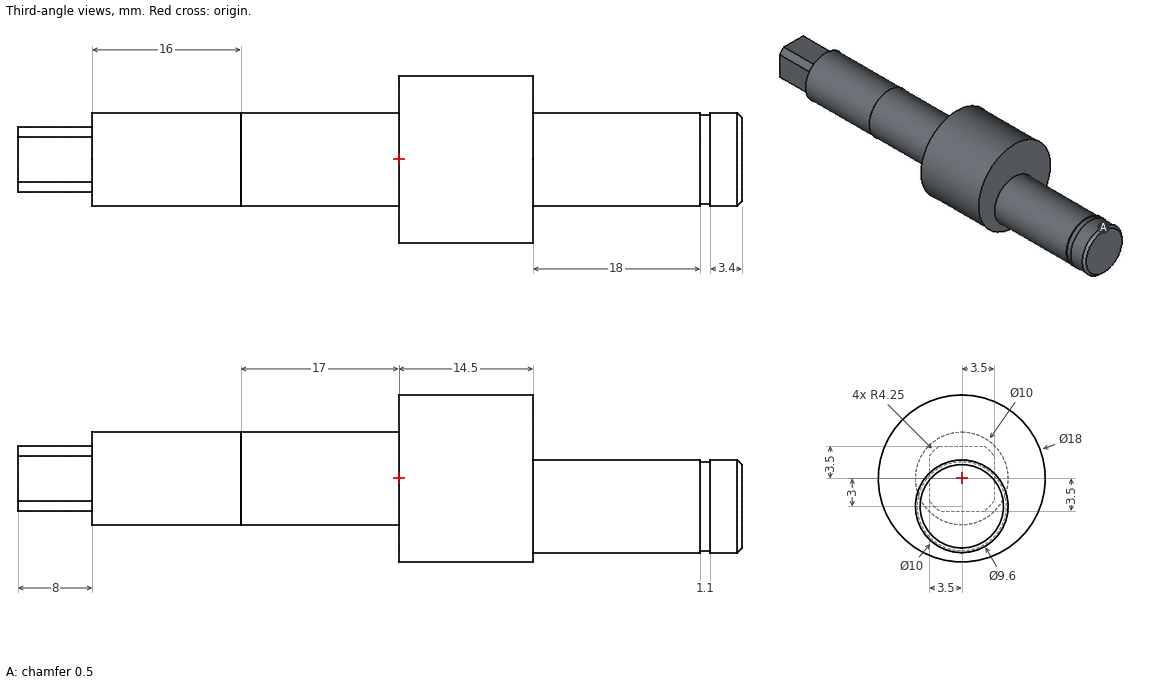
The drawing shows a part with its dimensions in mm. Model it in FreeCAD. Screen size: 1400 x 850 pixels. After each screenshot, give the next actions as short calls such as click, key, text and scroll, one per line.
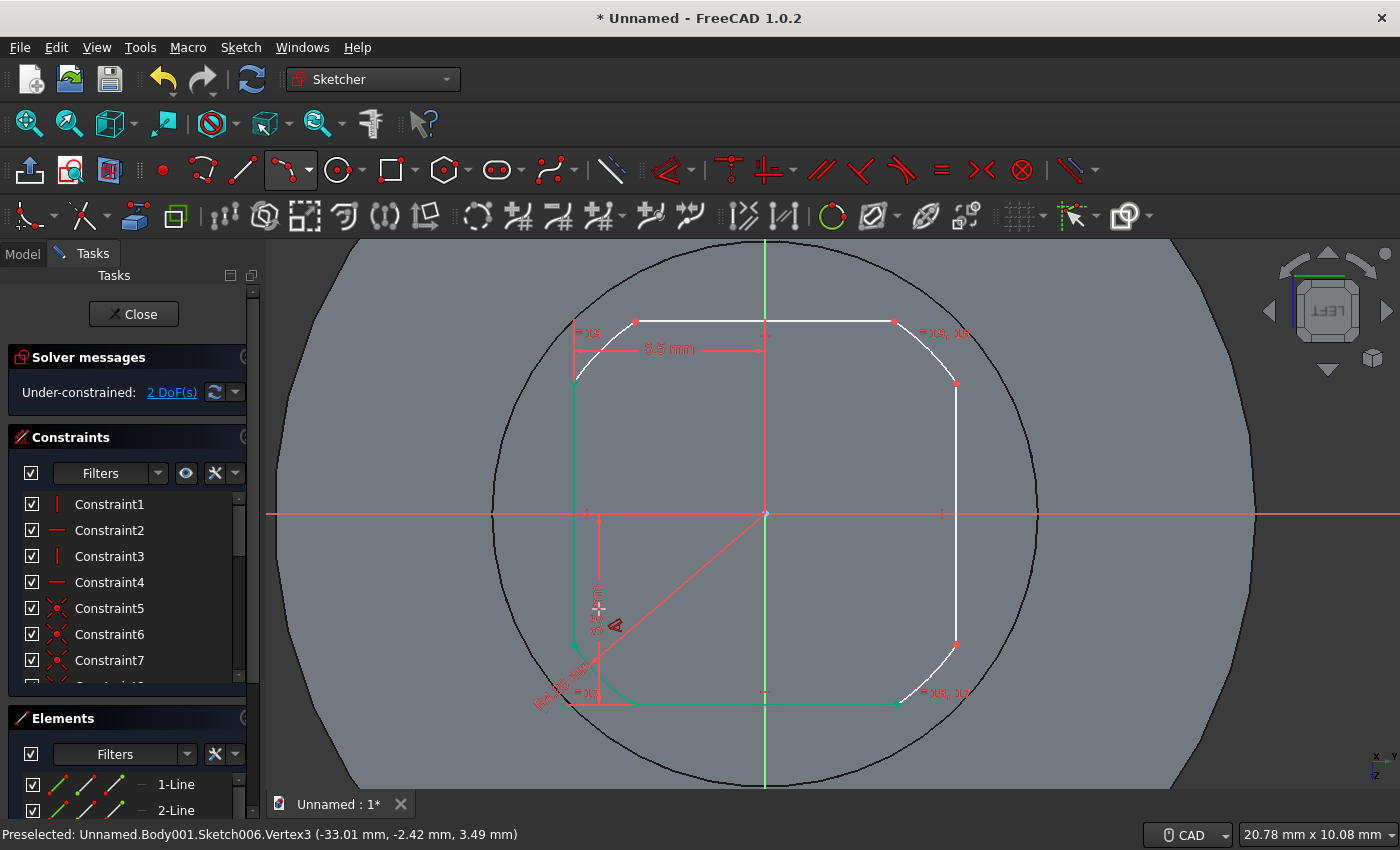
click(956, 645)
click(861, 679)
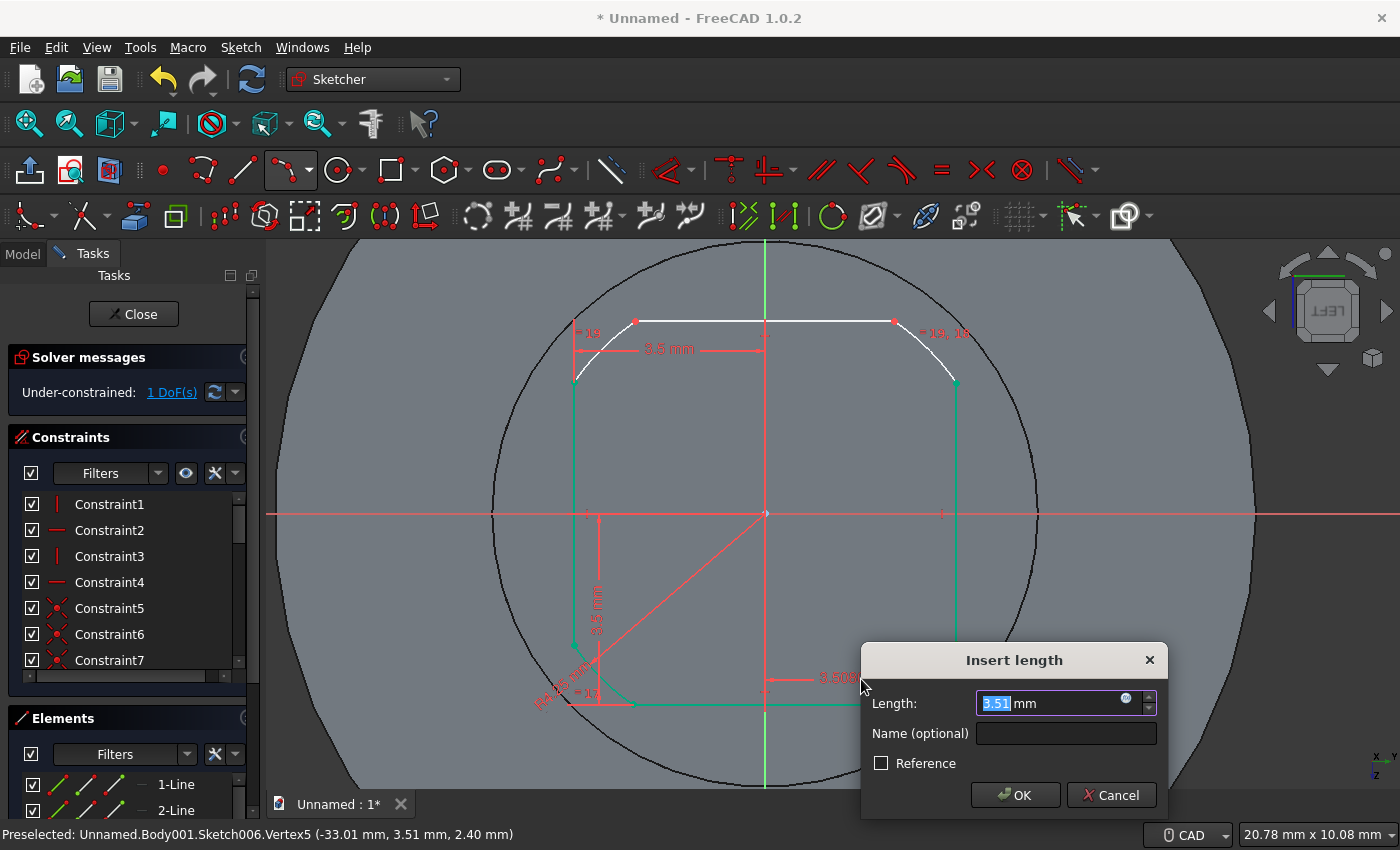
text(3.5)
key(Return)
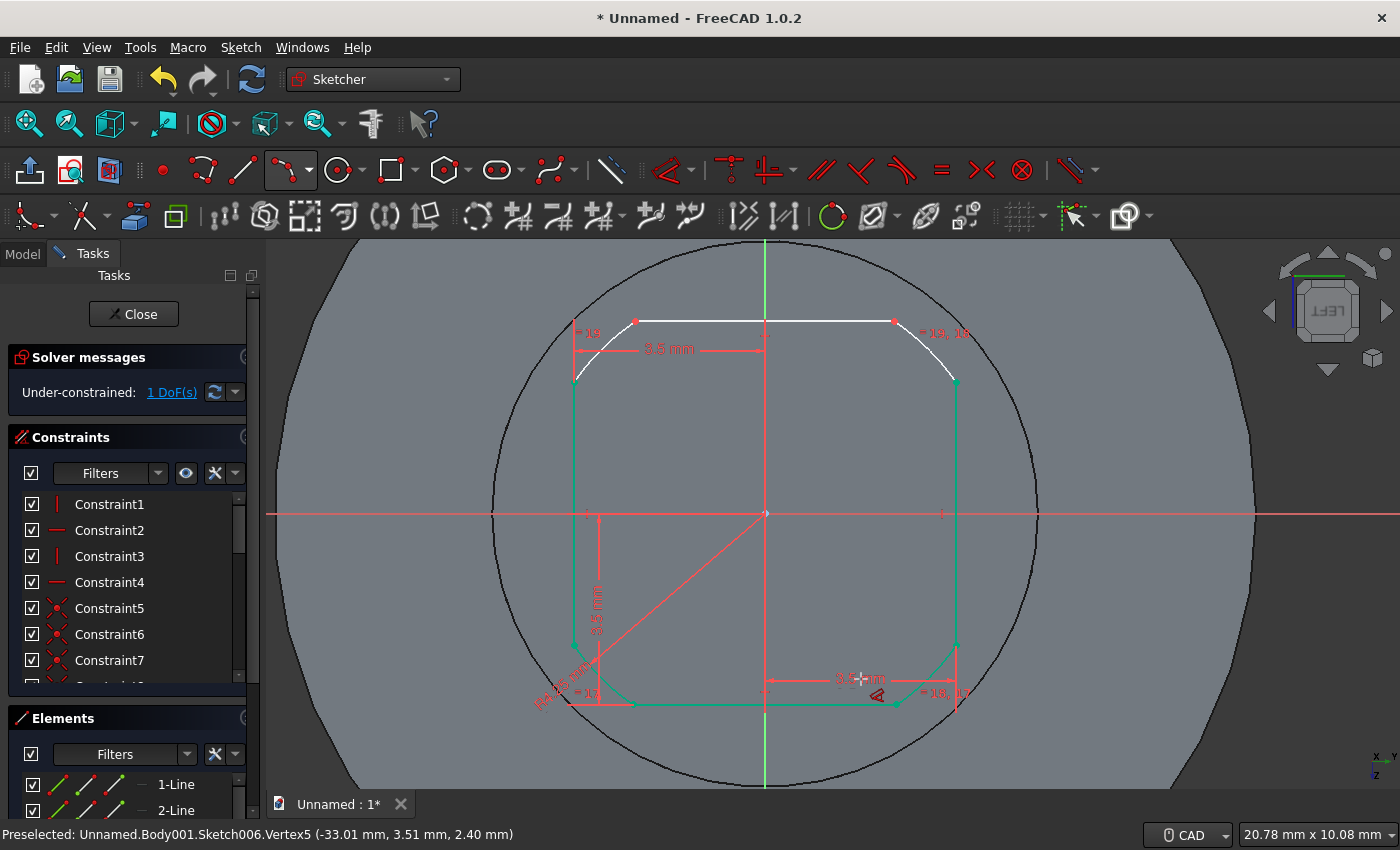
click(894, 321)
click(928, 418)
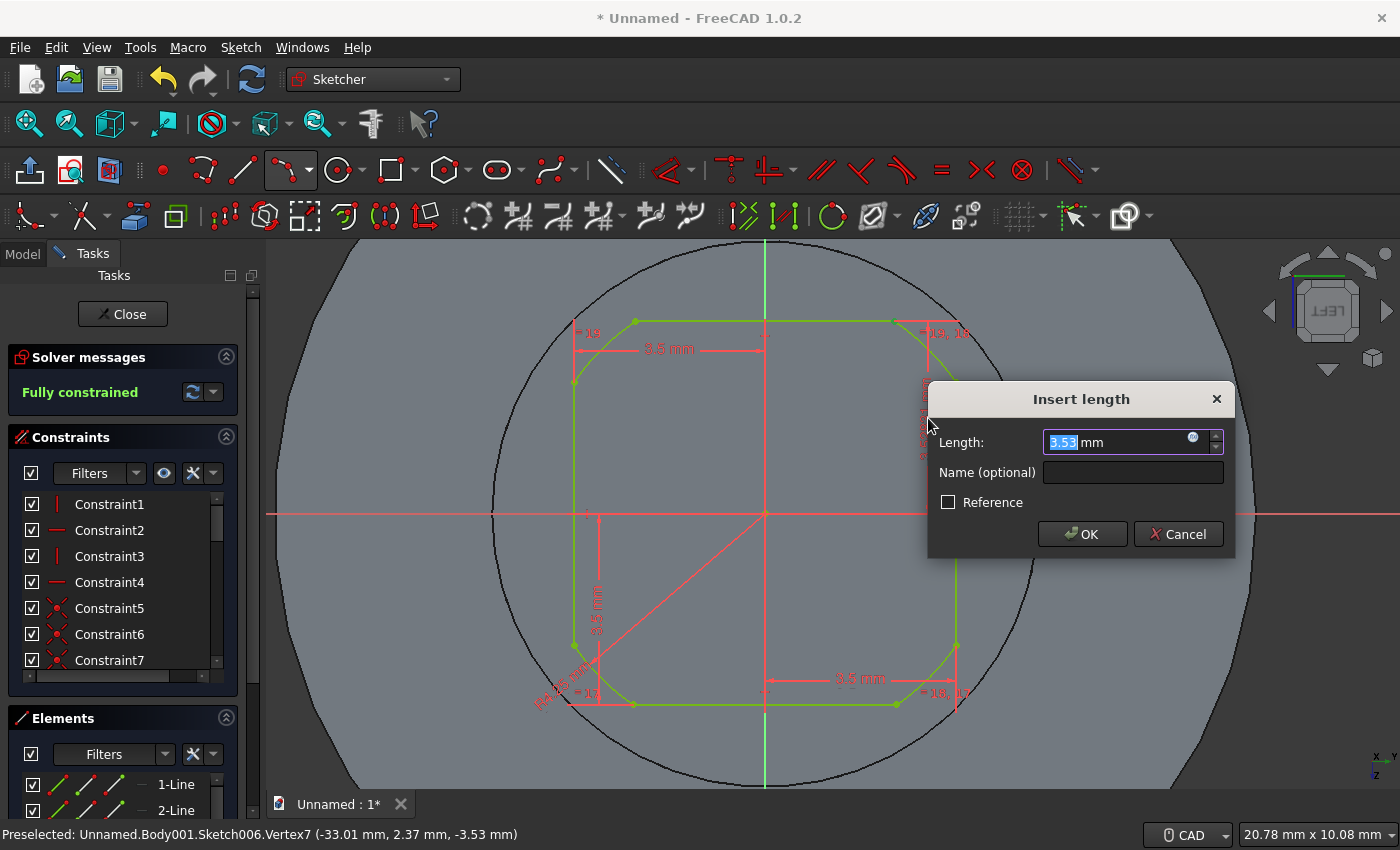
text(3.5)
key(Return)
key(Escape)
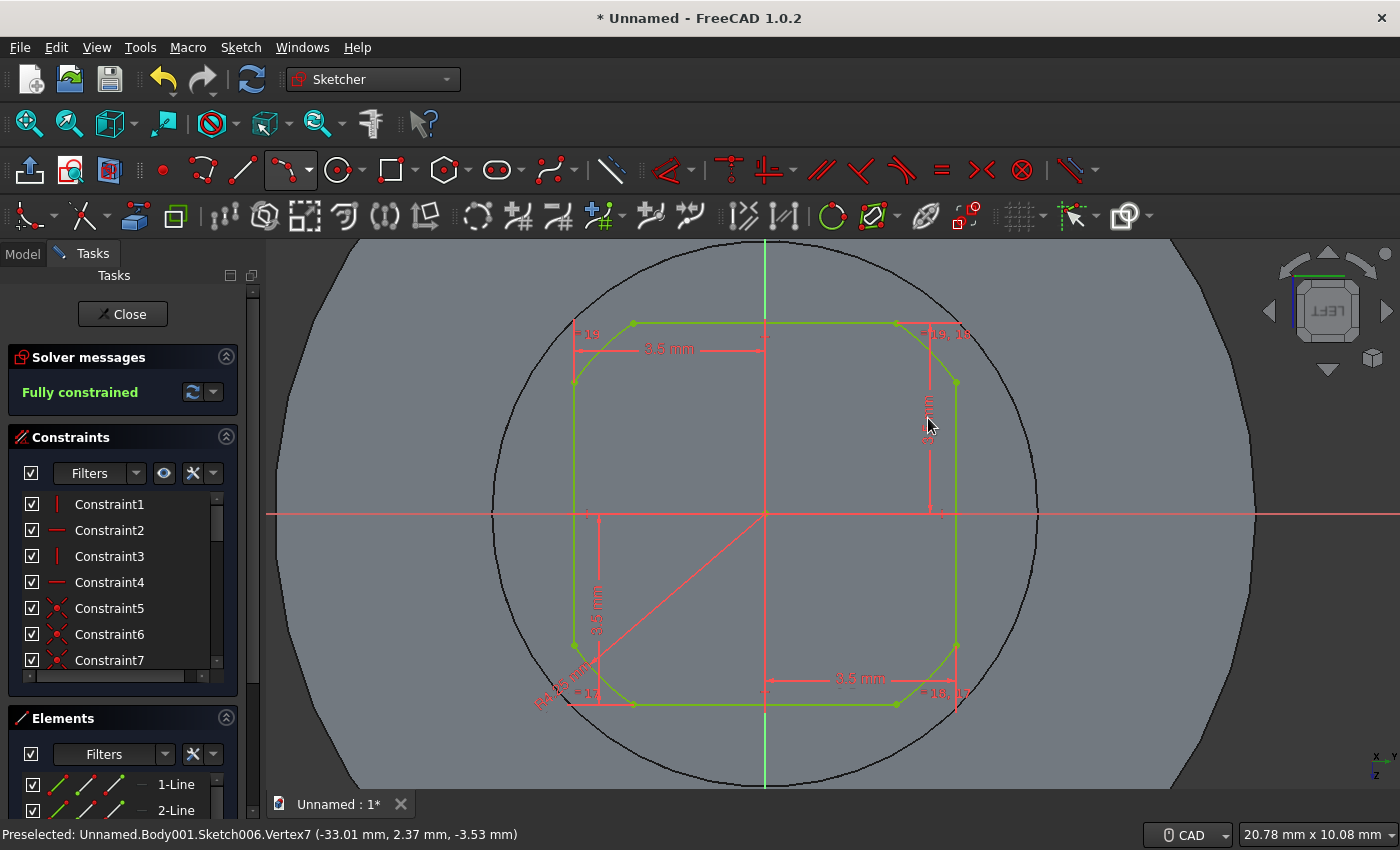
click(123, 314)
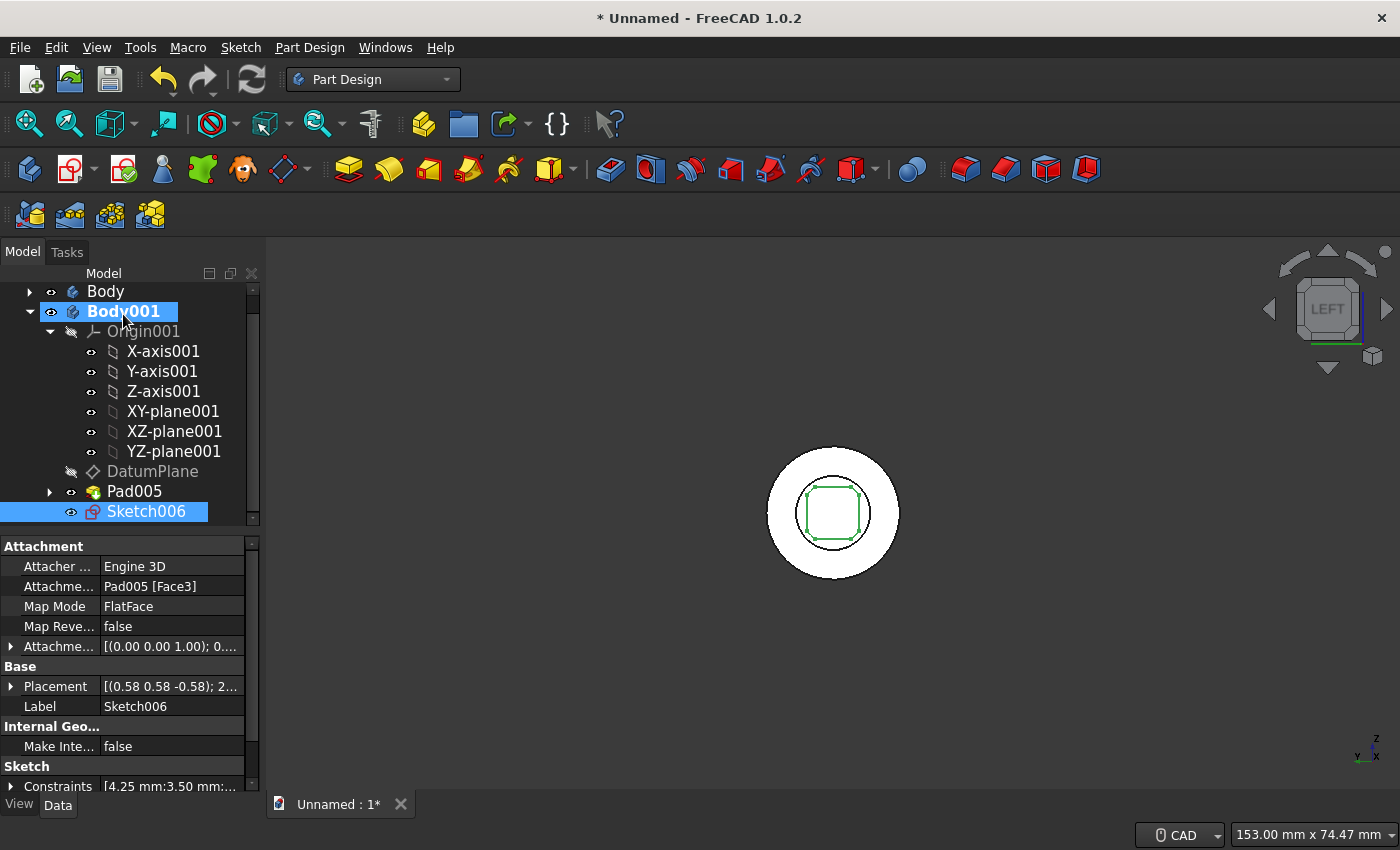
click(350, 170)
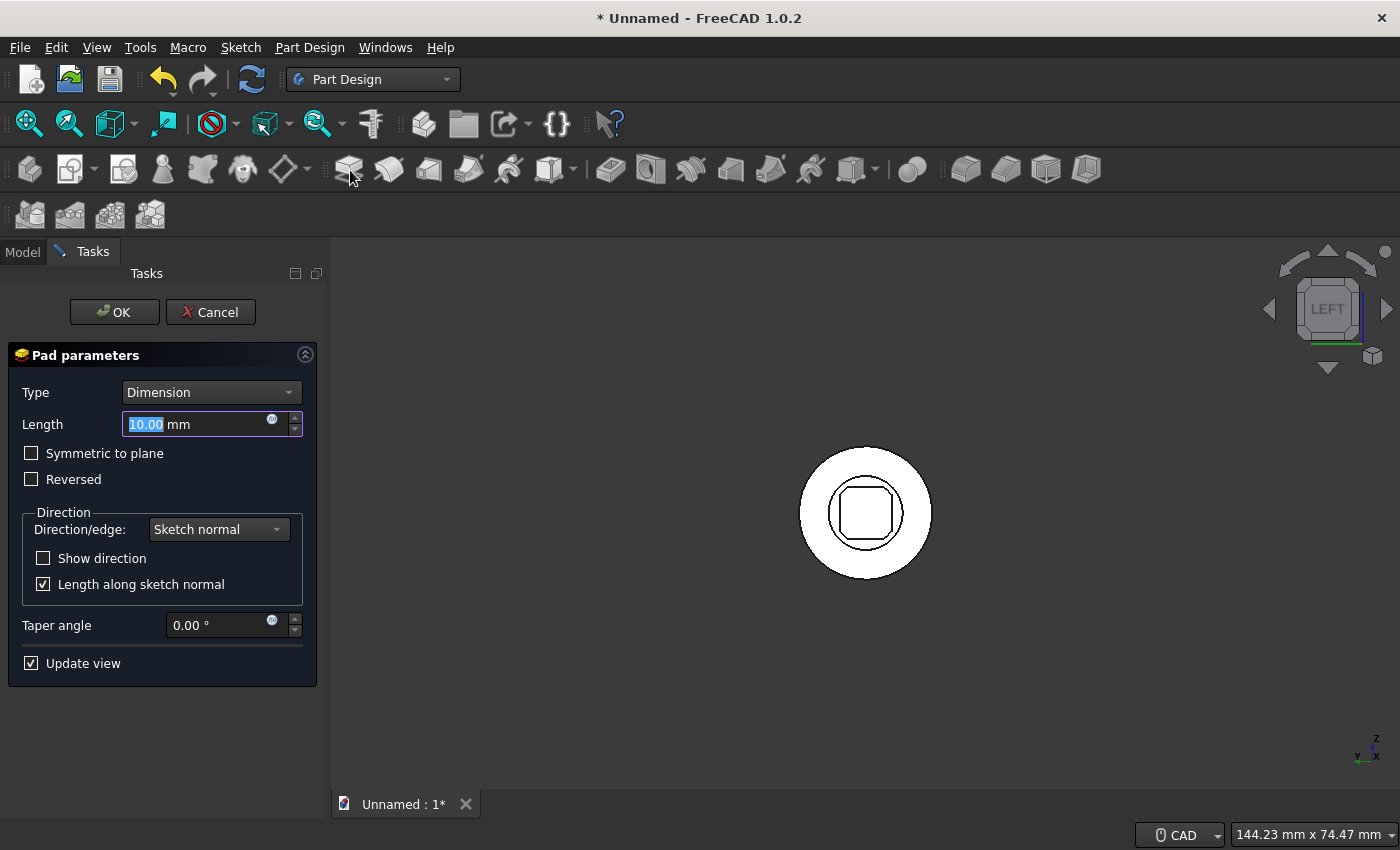
text(8)
key(Tab)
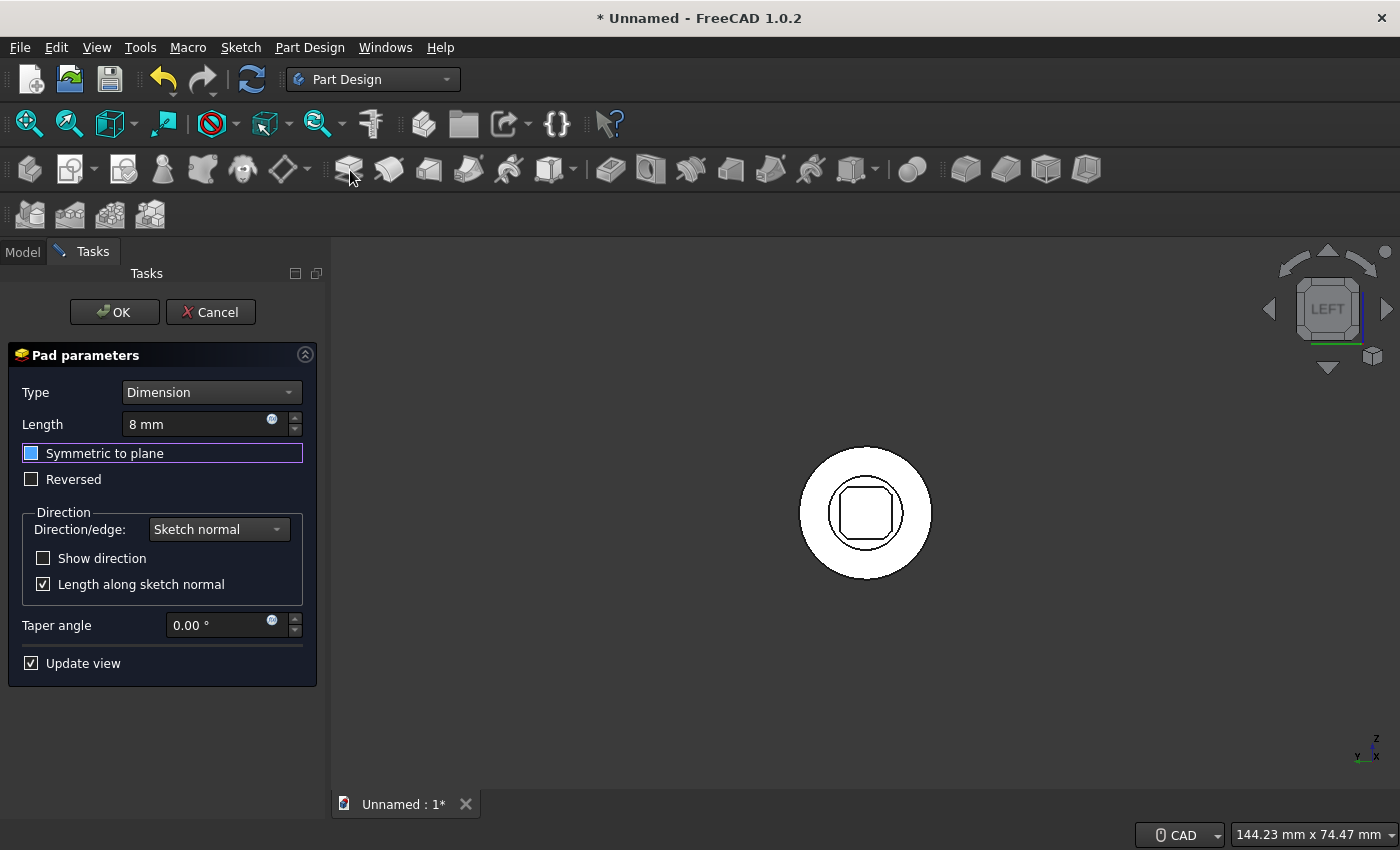
click(115, 312)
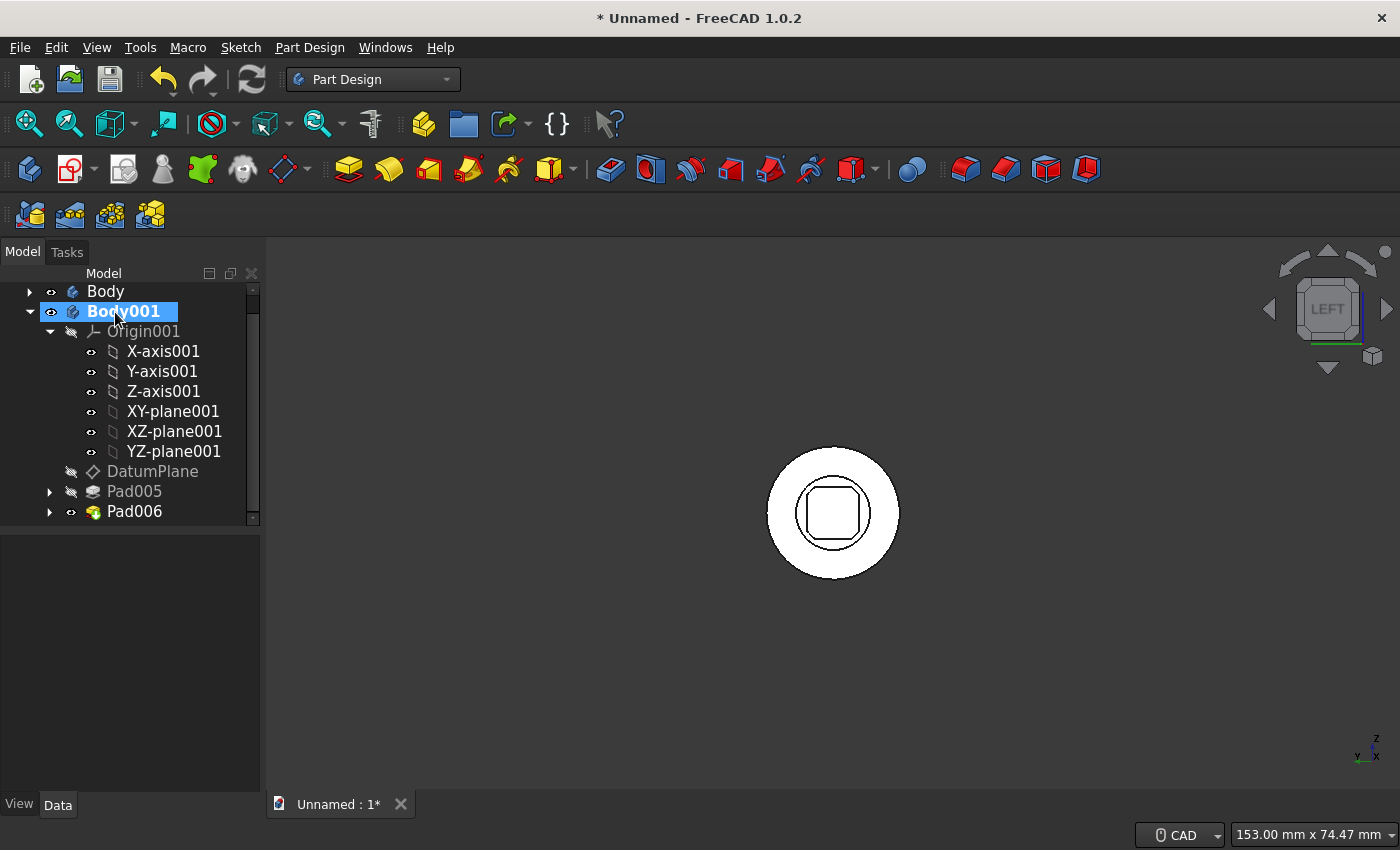
key(0)